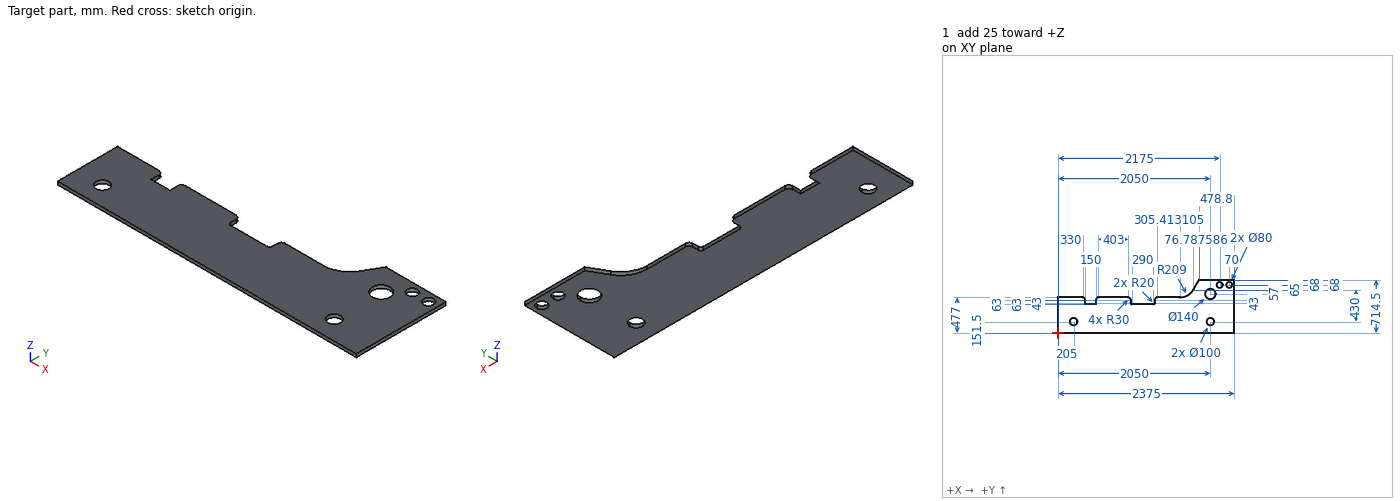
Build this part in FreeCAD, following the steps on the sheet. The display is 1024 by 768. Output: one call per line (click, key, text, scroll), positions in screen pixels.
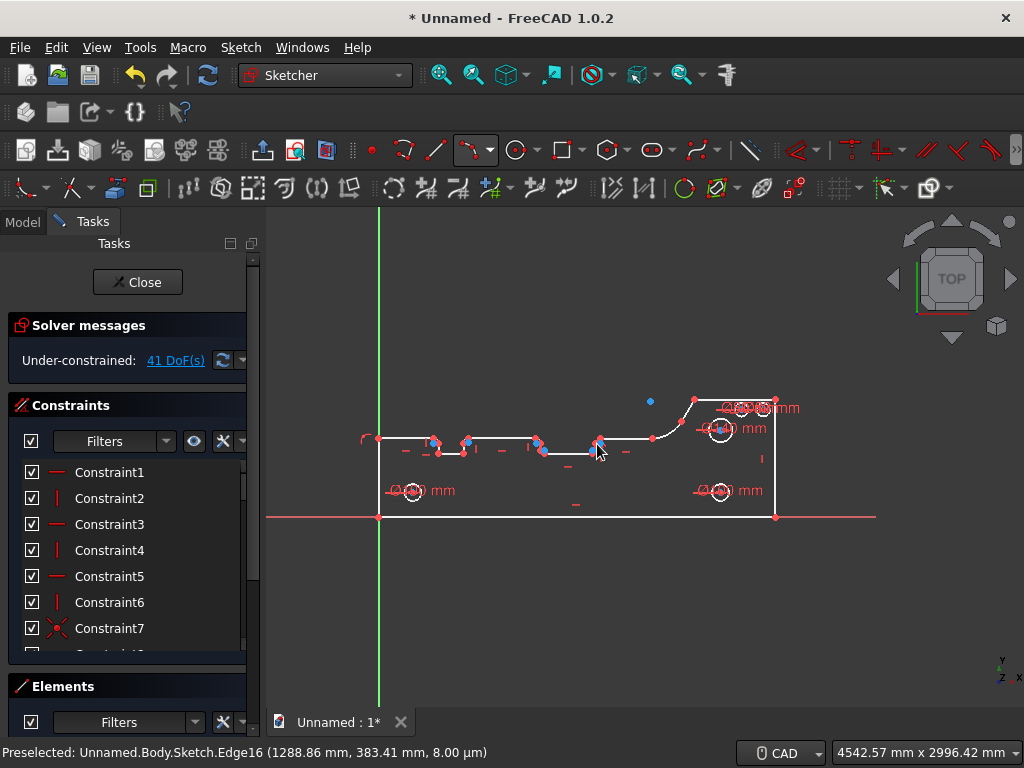
click(578, 454)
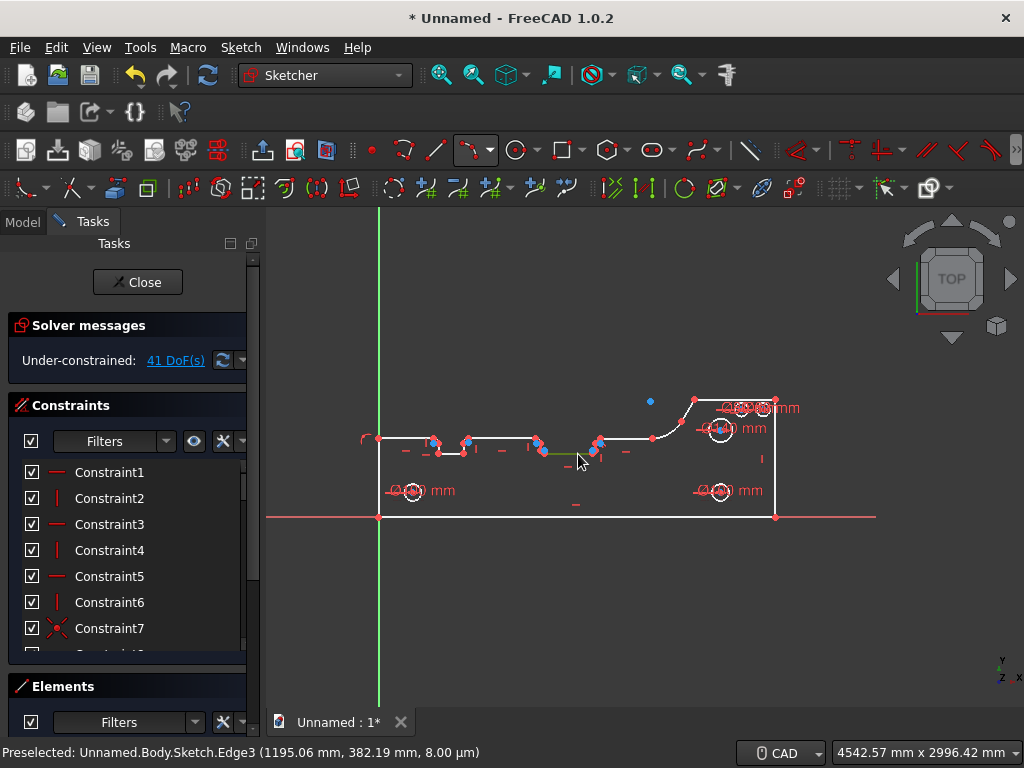
scroll(595, 453, up, 9)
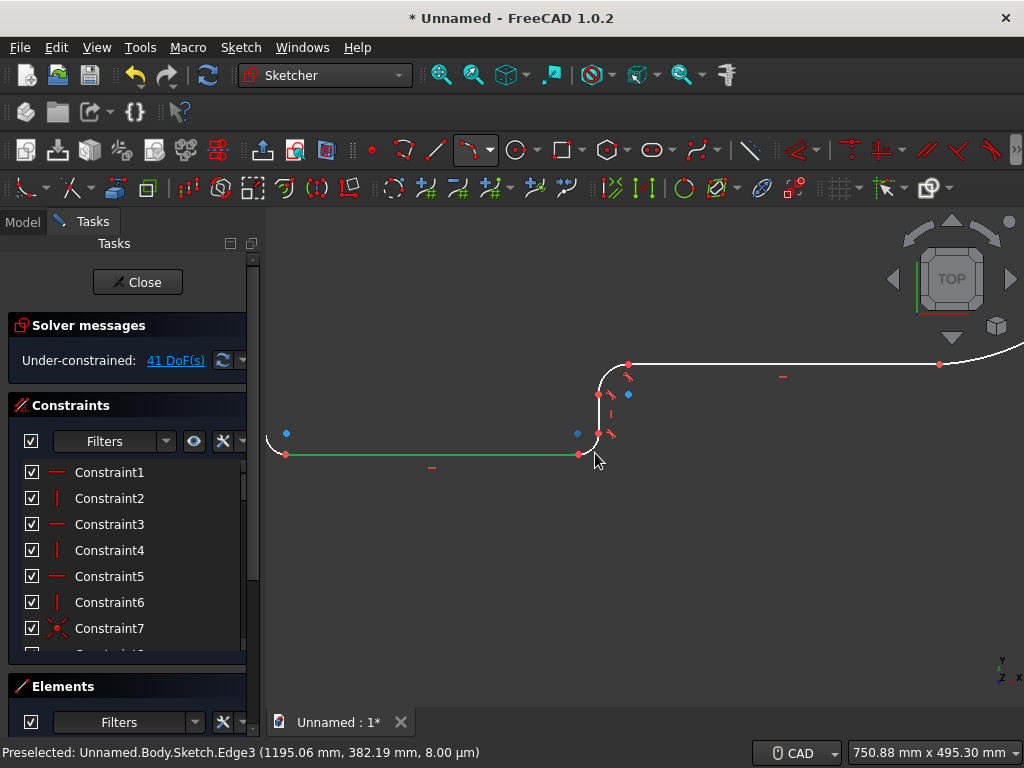
click(593, 448)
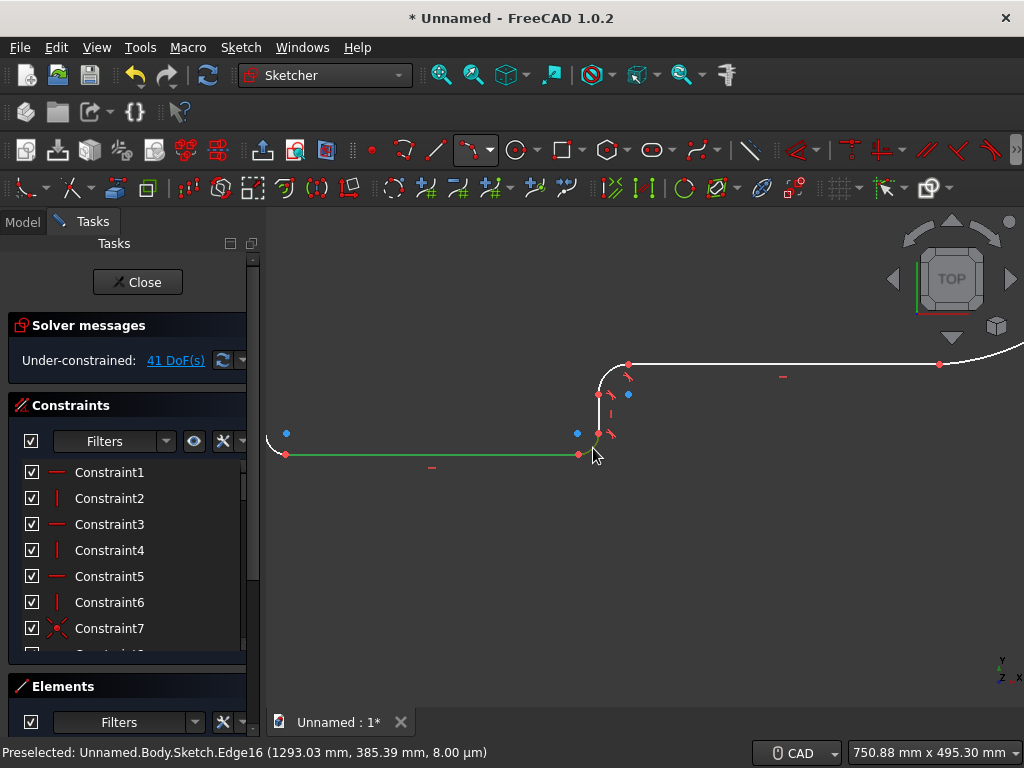
click(992, 150)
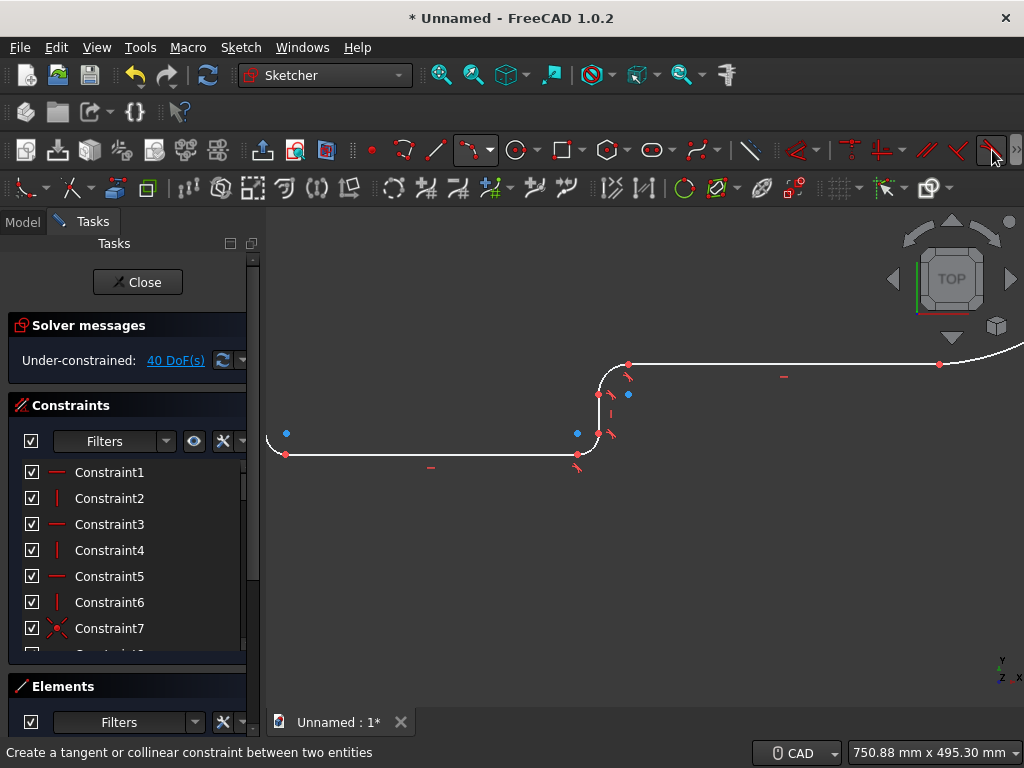
scroll(595, 452, down, 9)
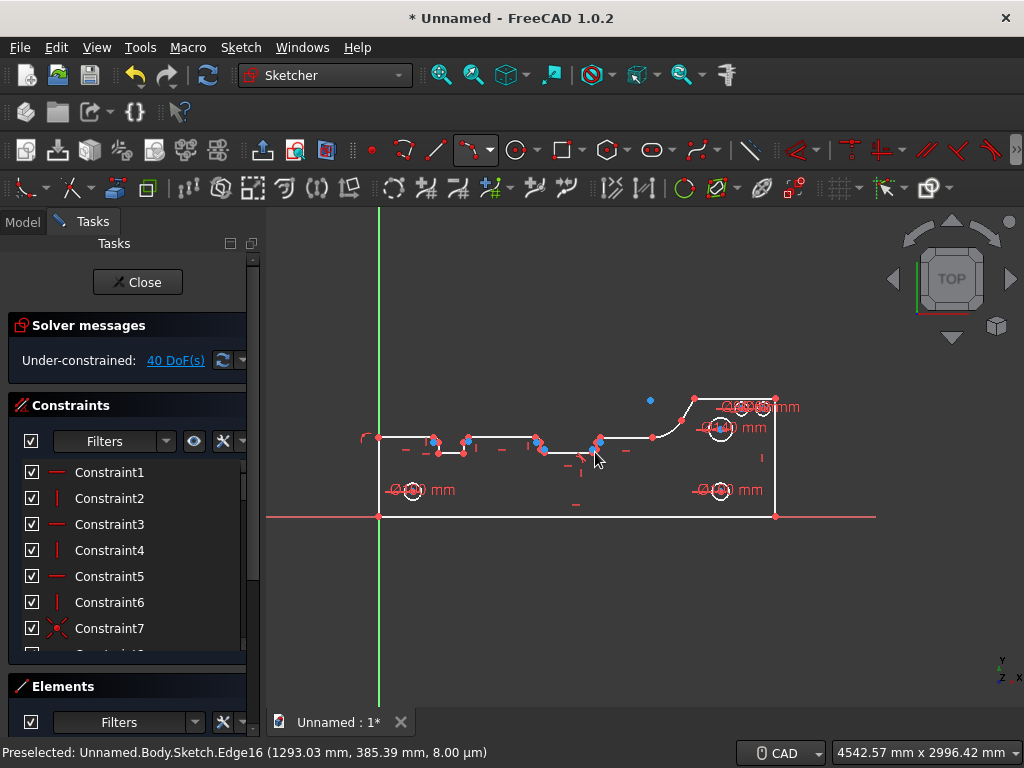
click(559, 453)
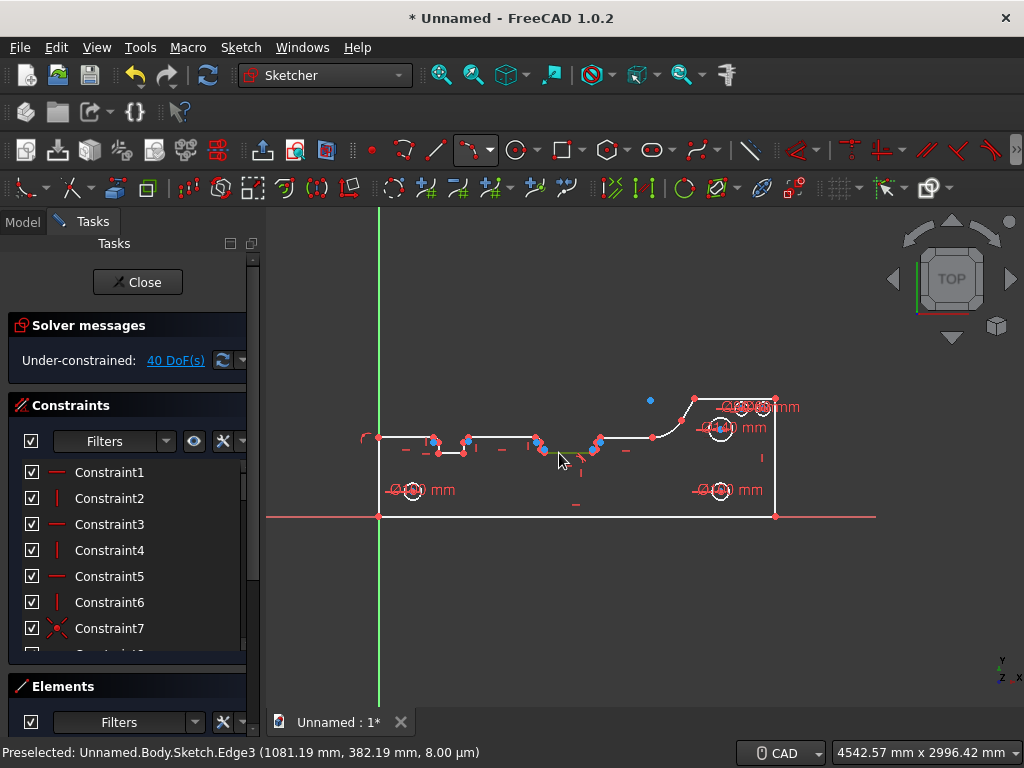
scroll(542, 452, up, 9)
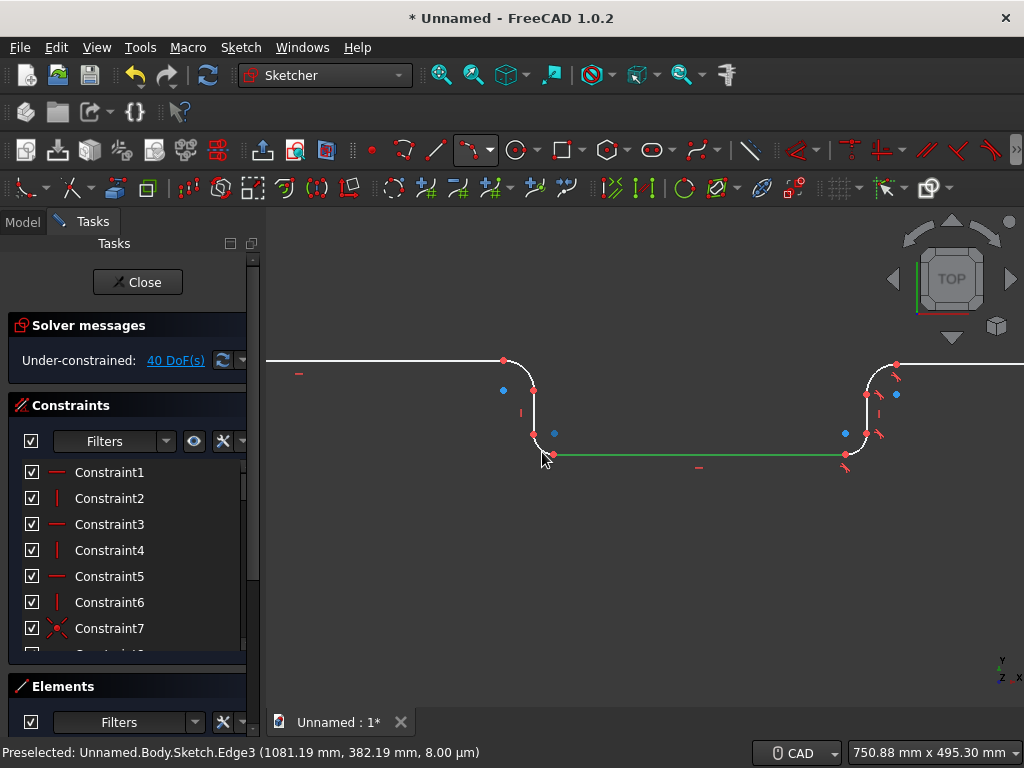
click(540, 449)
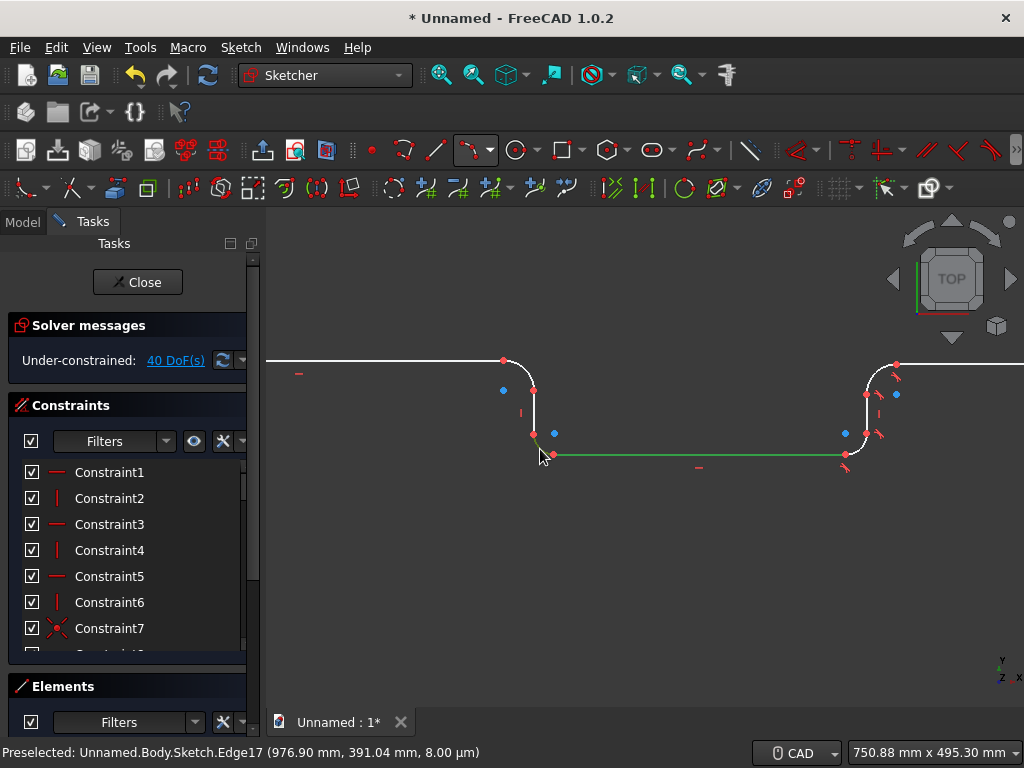
click(992, 150)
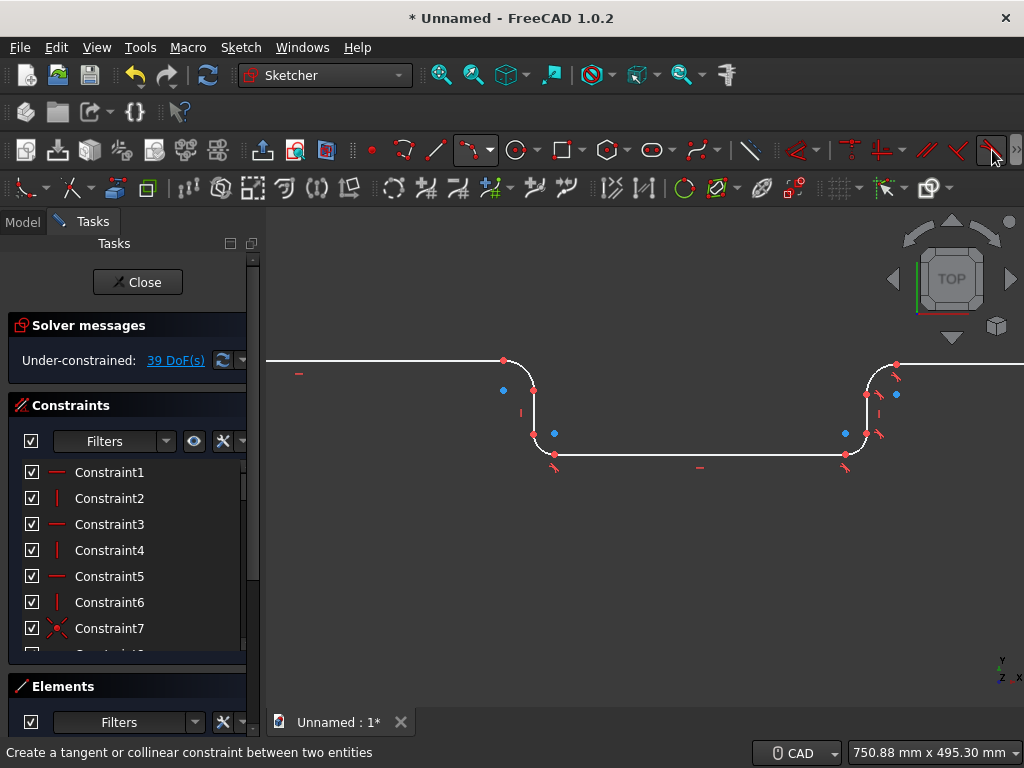
click(534, 422)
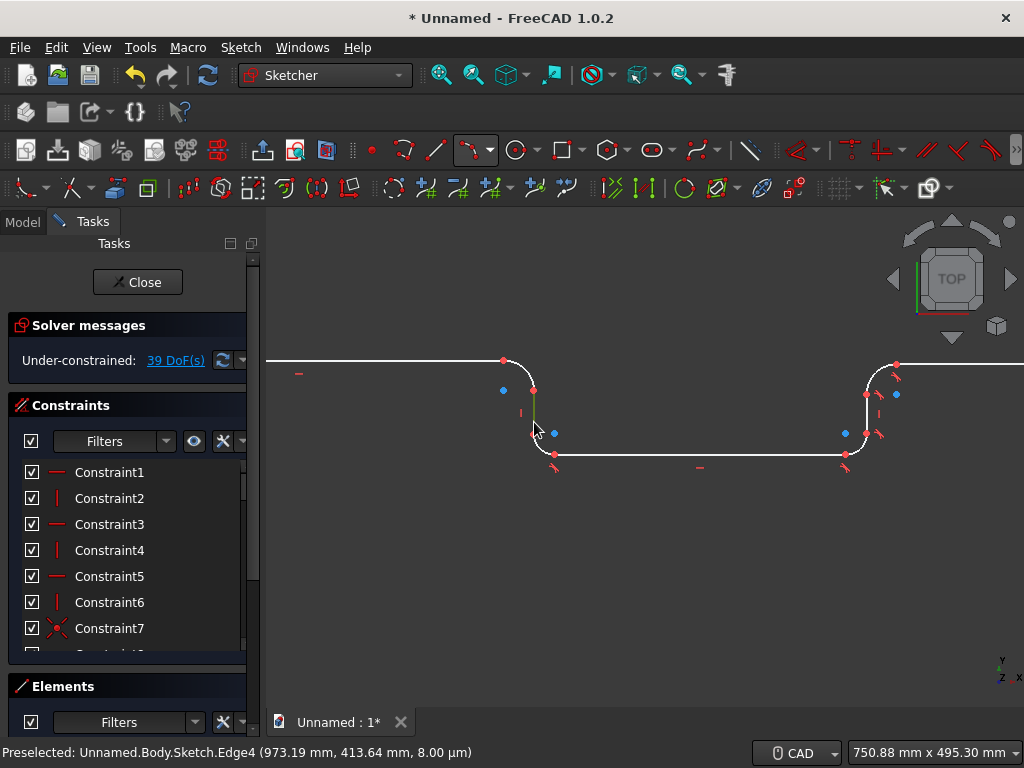
scroll(537, 444, up, 2)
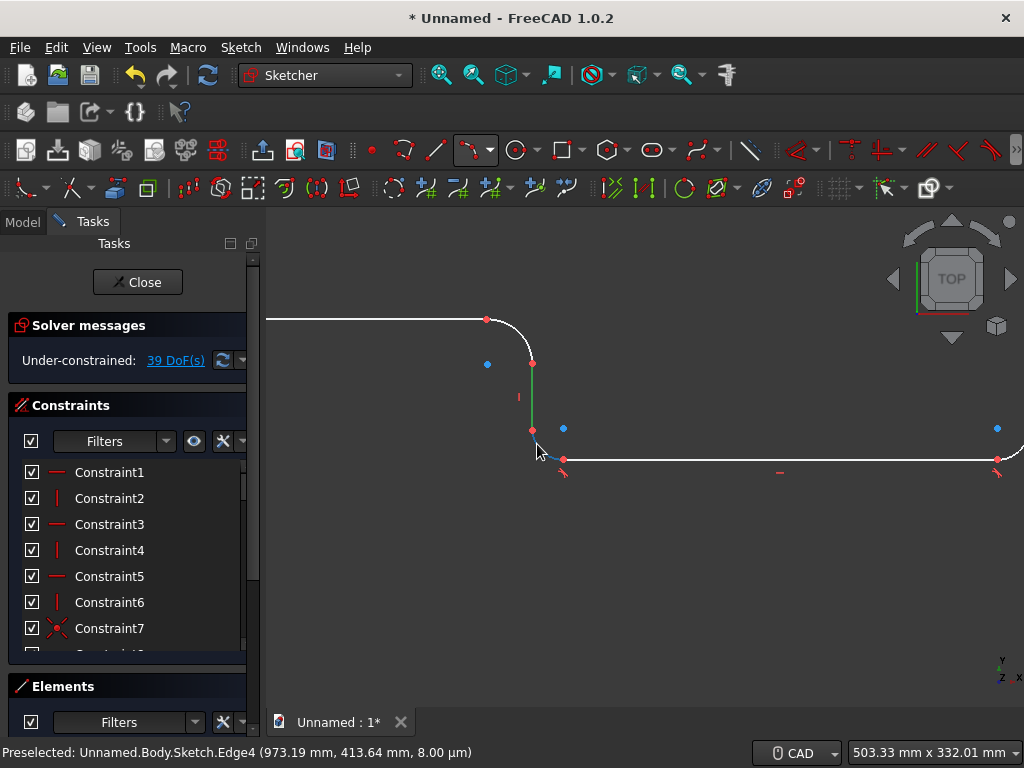
click(536, 444)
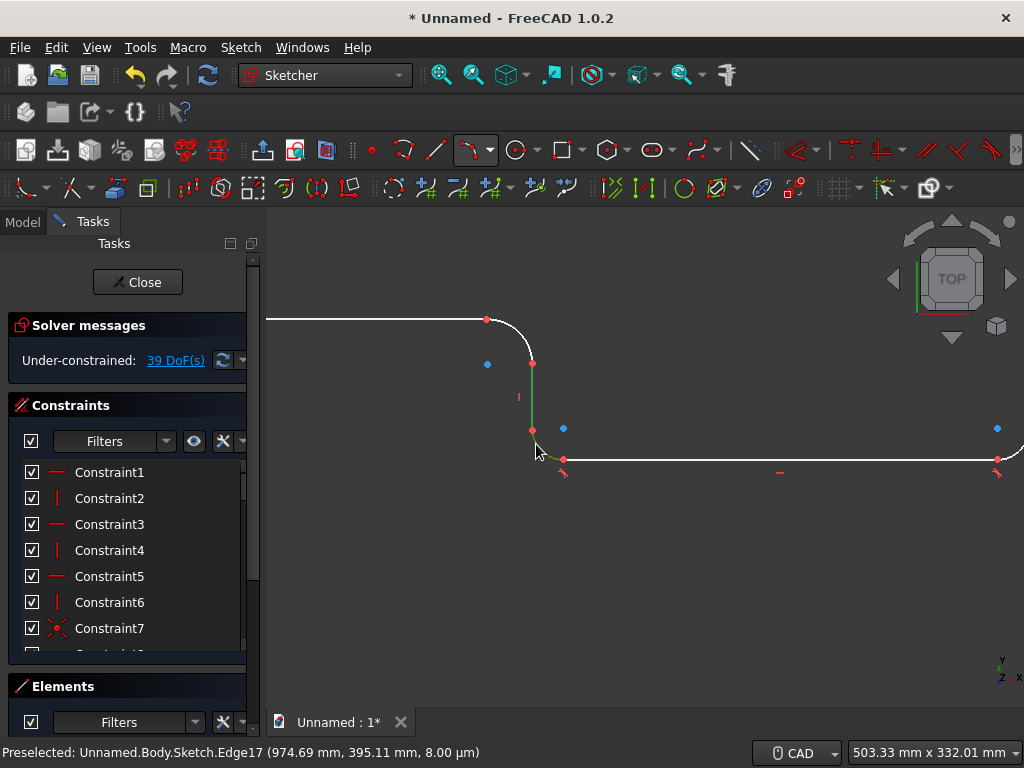
click(992, 150)